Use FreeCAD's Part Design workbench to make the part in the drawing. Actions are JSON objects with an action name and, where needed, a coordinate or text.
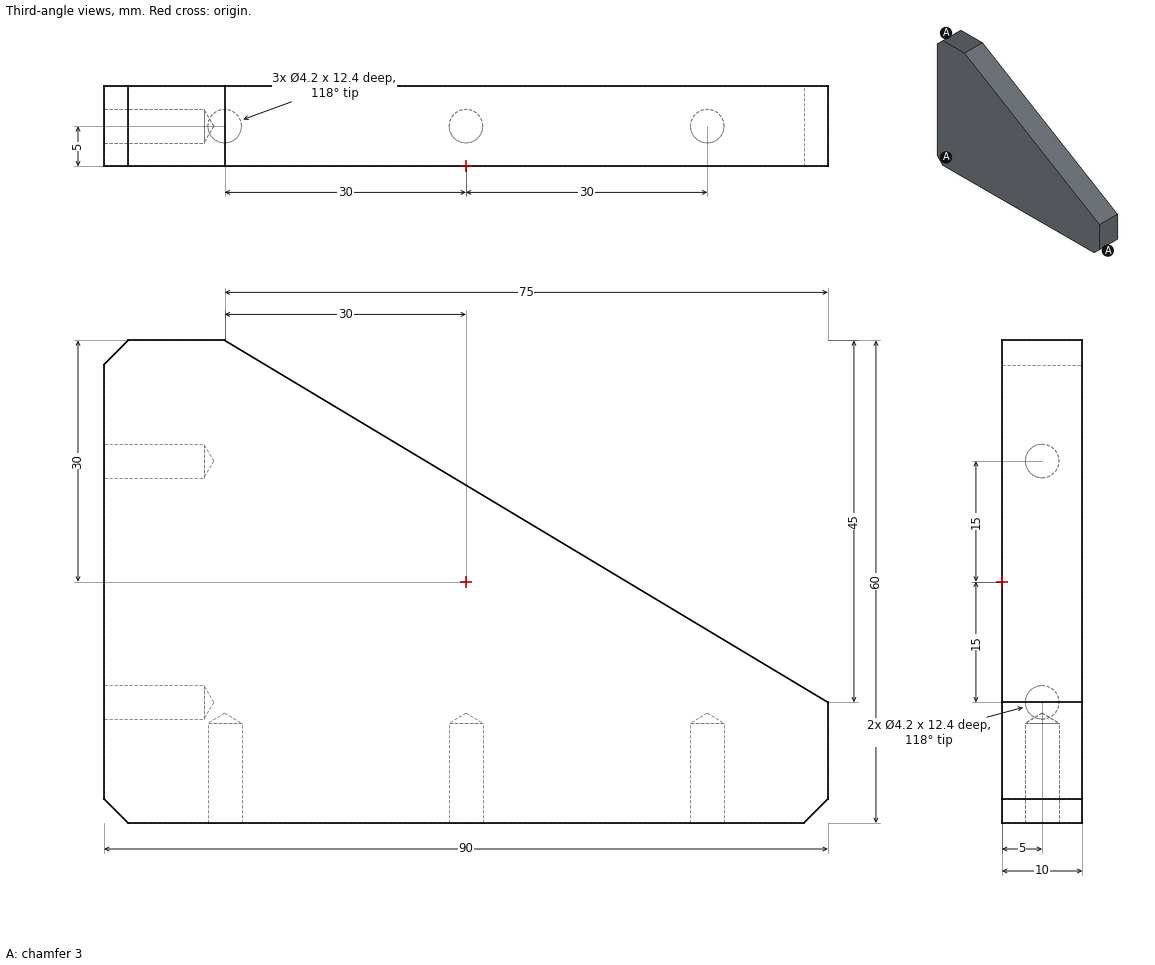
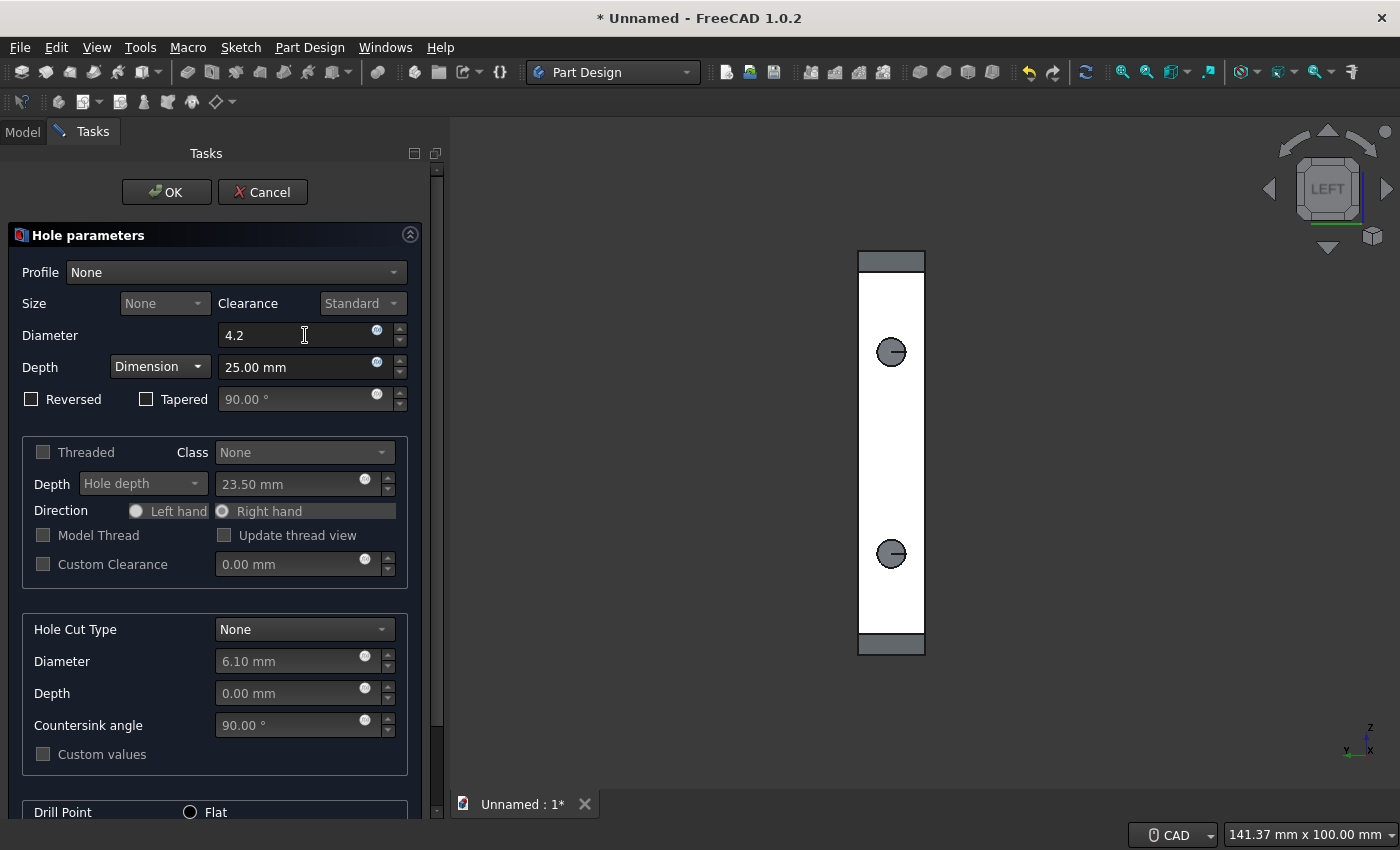
{"action": "triple_click", "coordinate": [305, 367]}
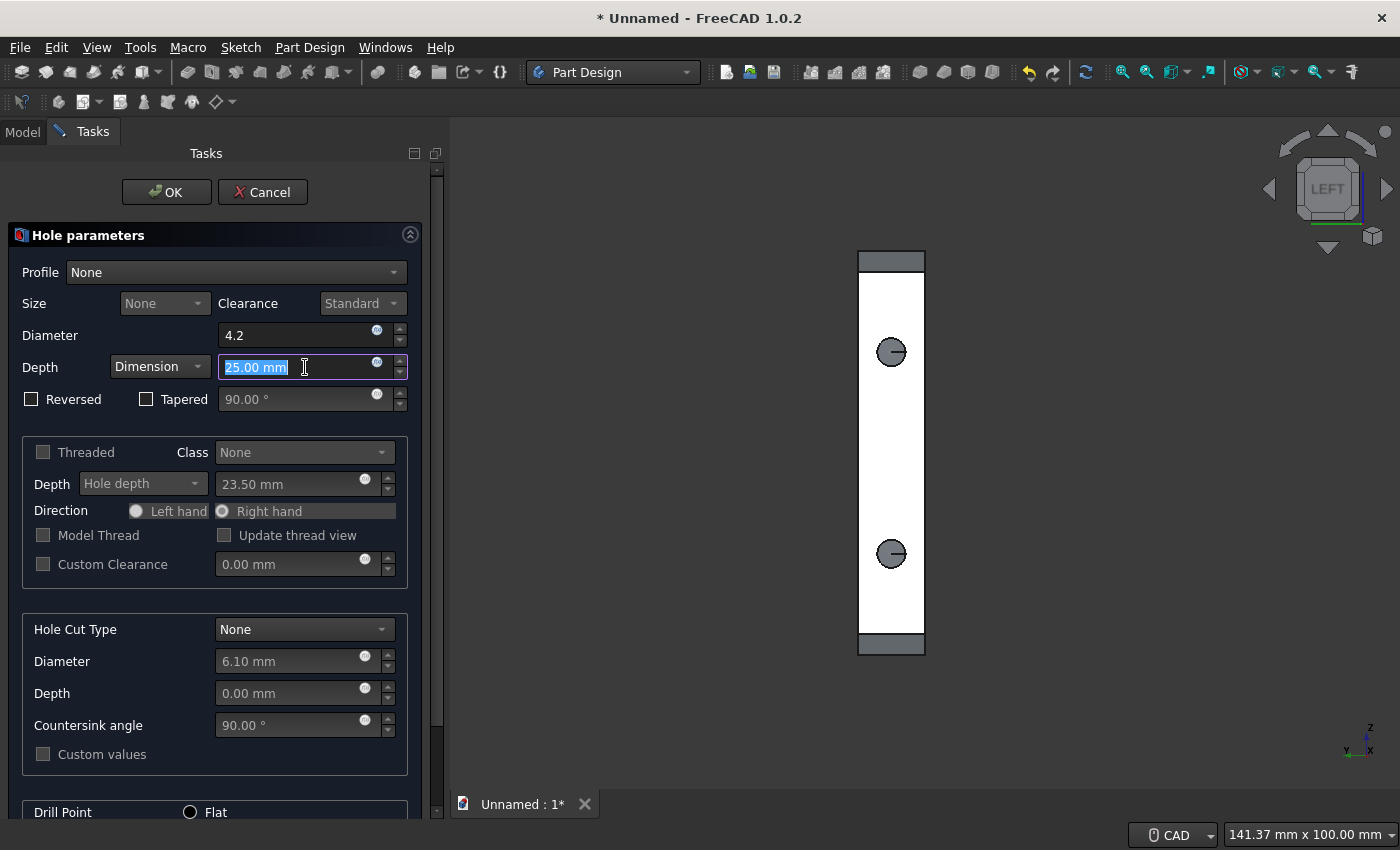
{"action": "type", "text": "12.4"}
{"action": "key", "text": "Tab"}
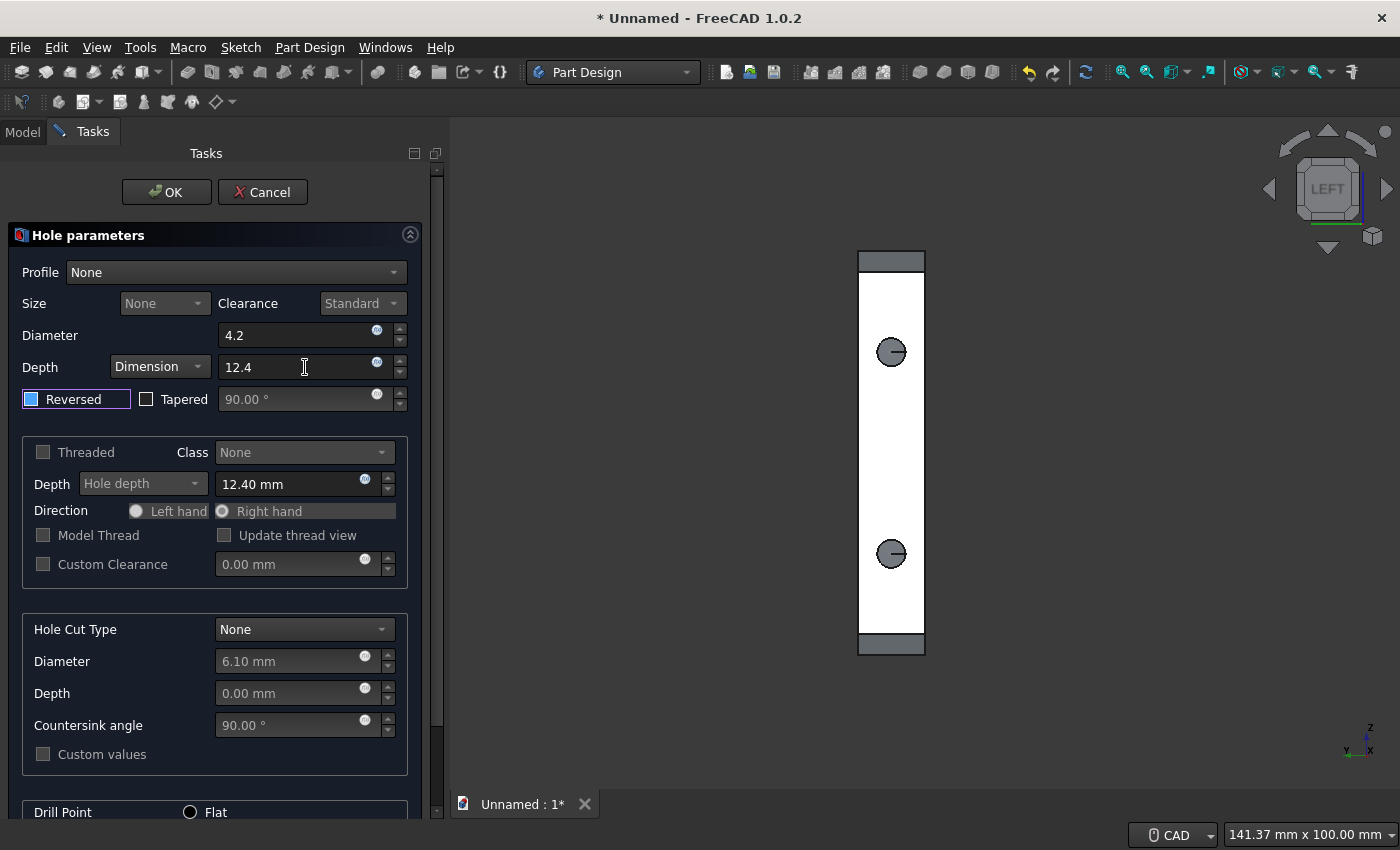
{"action": "left_click", "coordinate": [167, 192]}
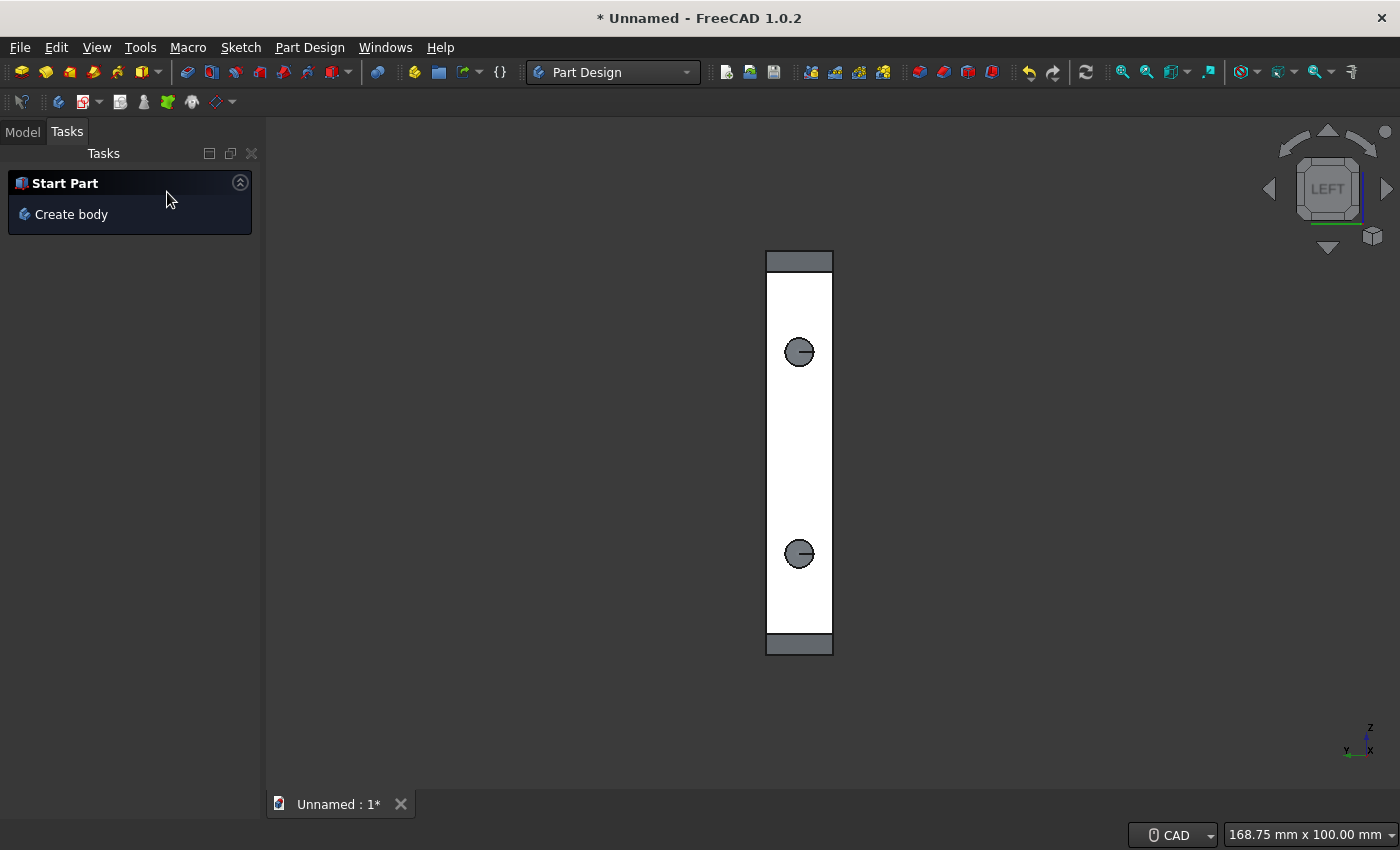
{"action": "key", "text": "5"}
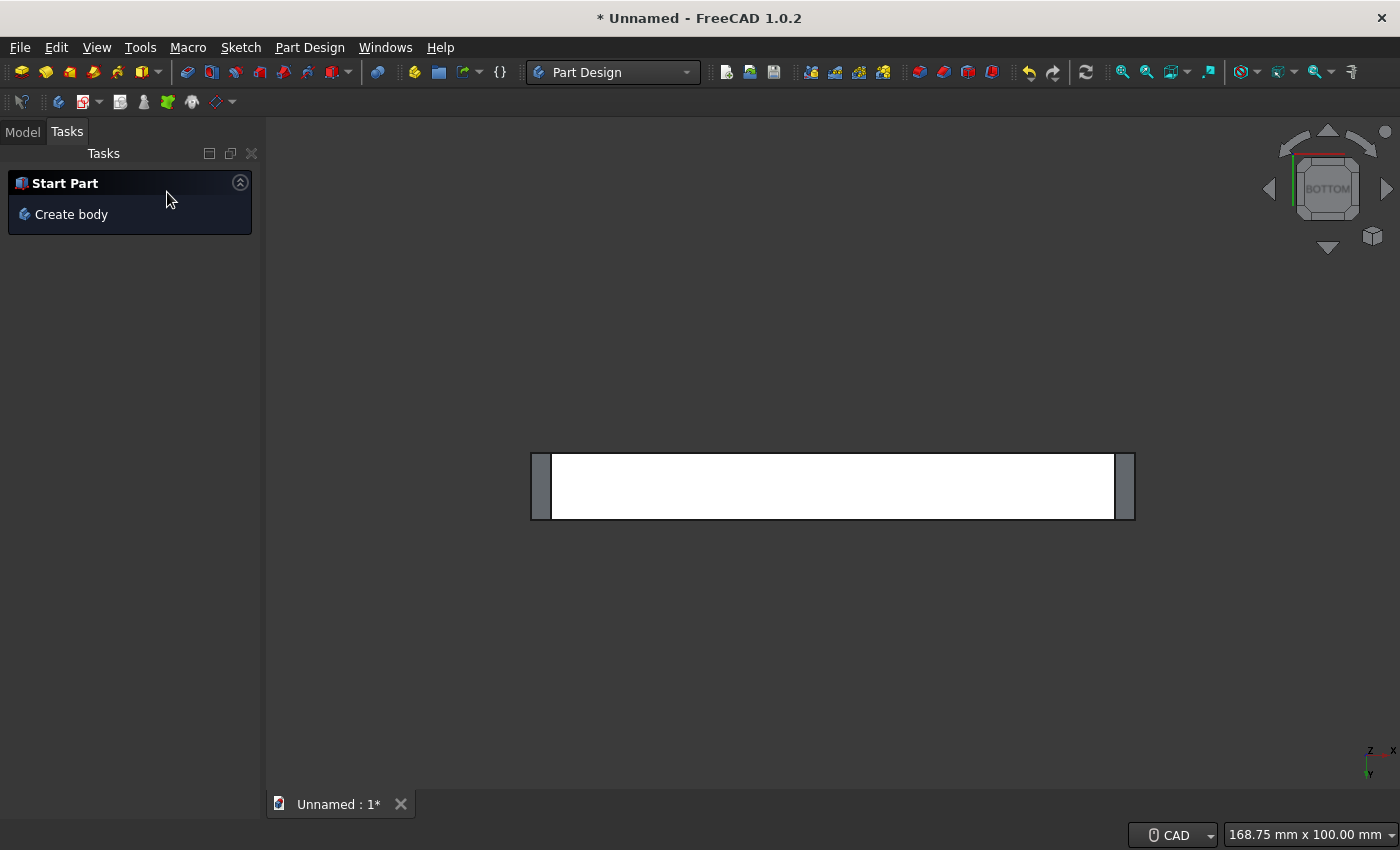
{"action": "left_click", "coordinate": [1075, 486]}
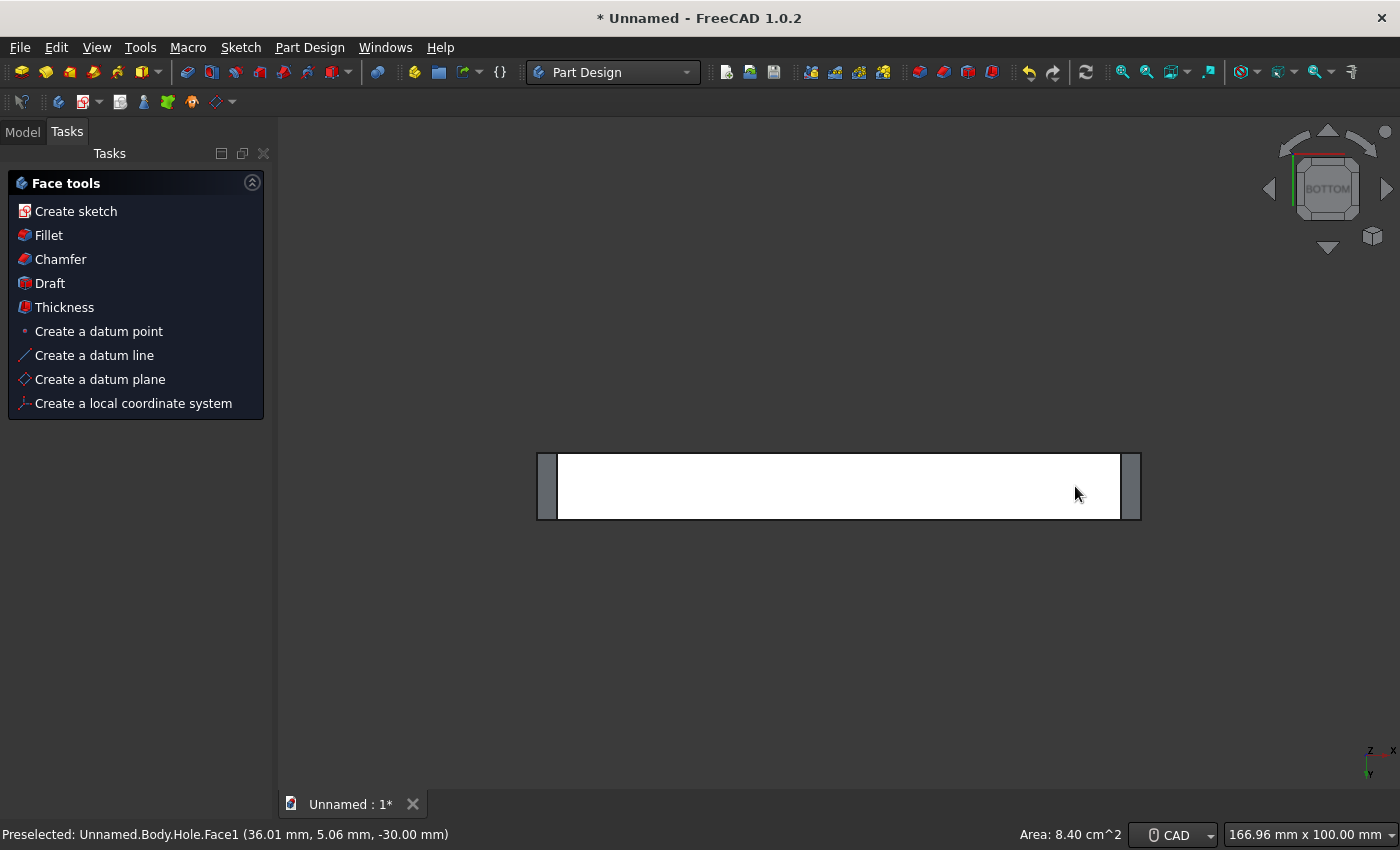
{"action": "left_click", "coordinate": [84, 102]}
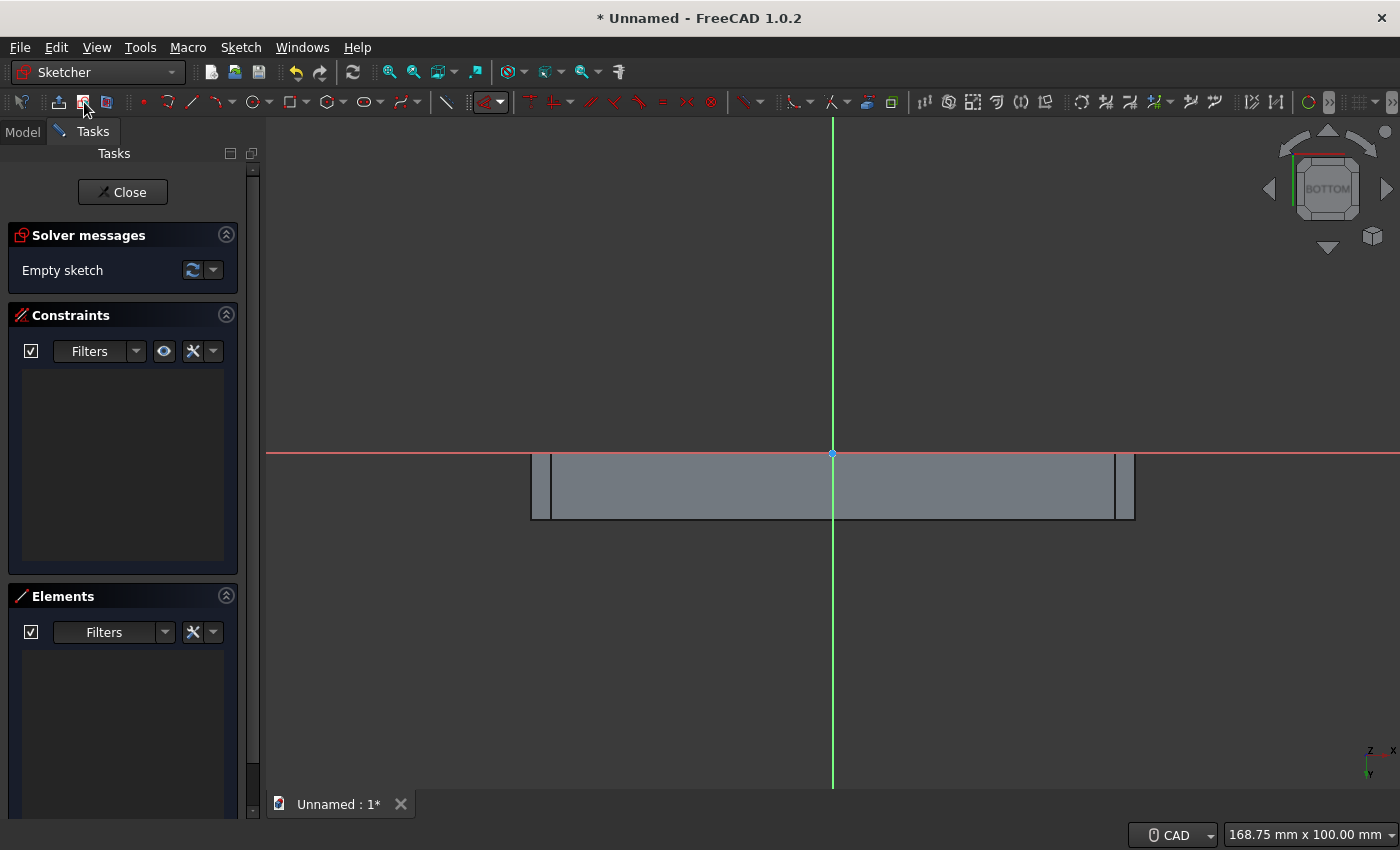
{"action": "scroll", "coordinate": [972, 525], "scroll_direction": "up", "scroll_amount": 2}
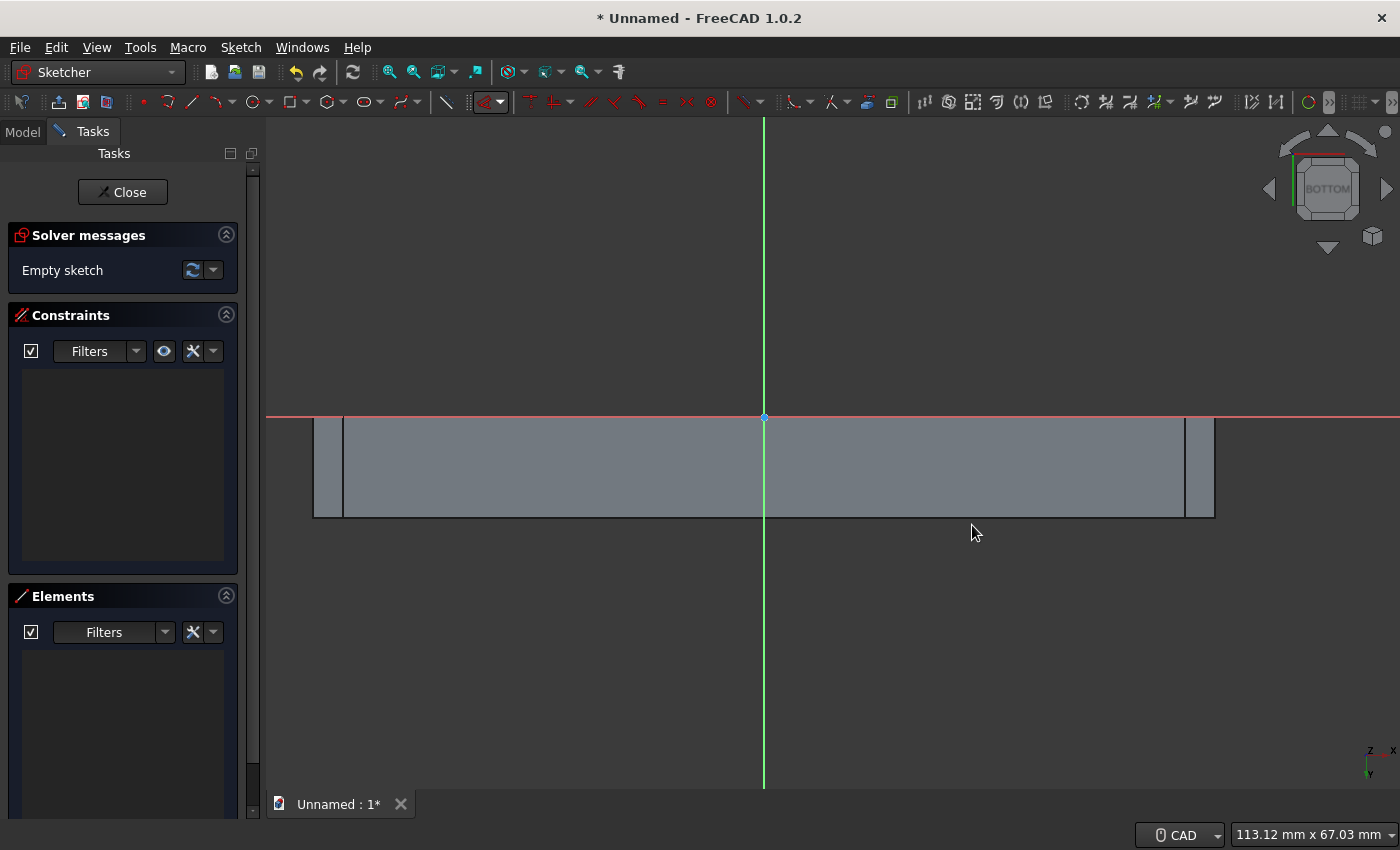
{"action": "key", "text": "g c"}